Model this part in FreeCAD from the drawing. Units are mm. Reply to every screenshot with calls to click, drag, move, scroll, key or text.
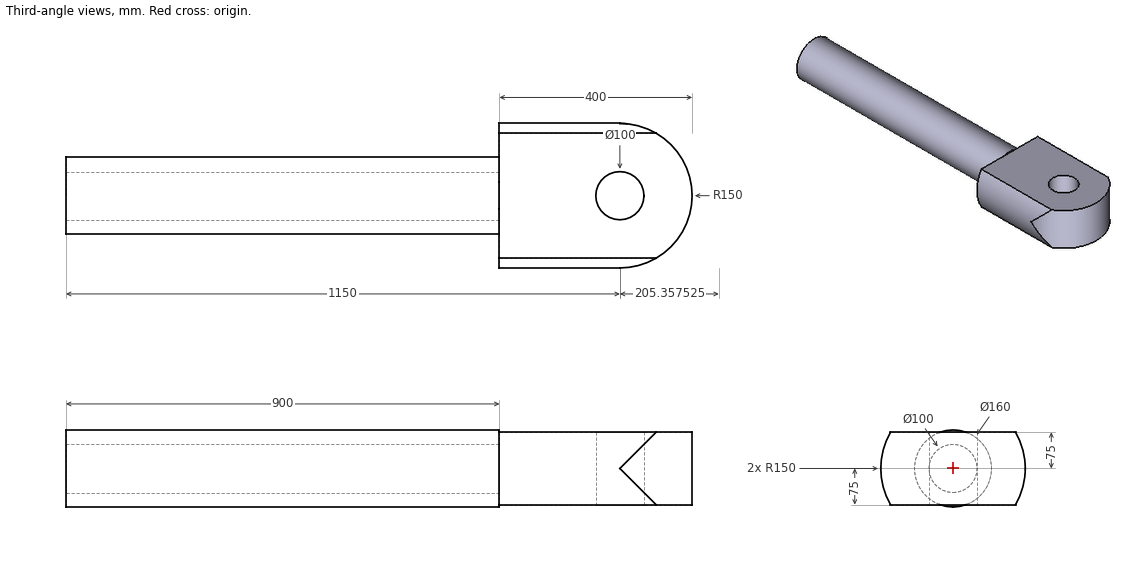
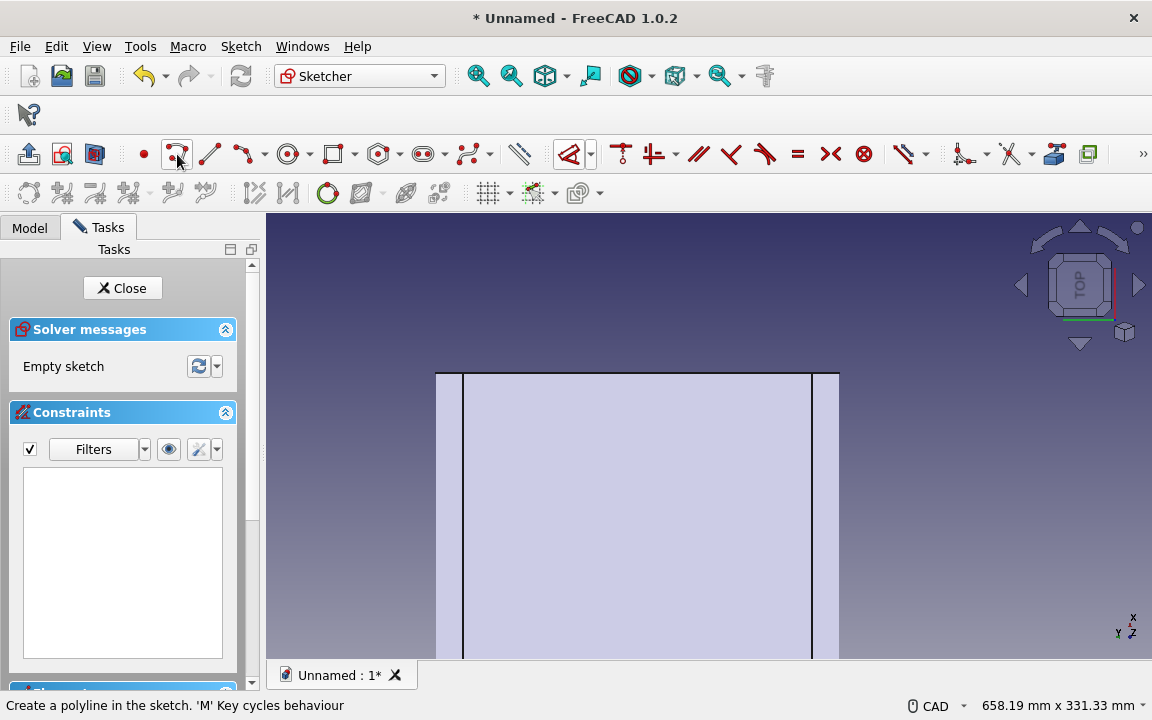
click(839, 575)
click(839, 299)
click(436, 299)
click(436, 575)
right_click(436, 575)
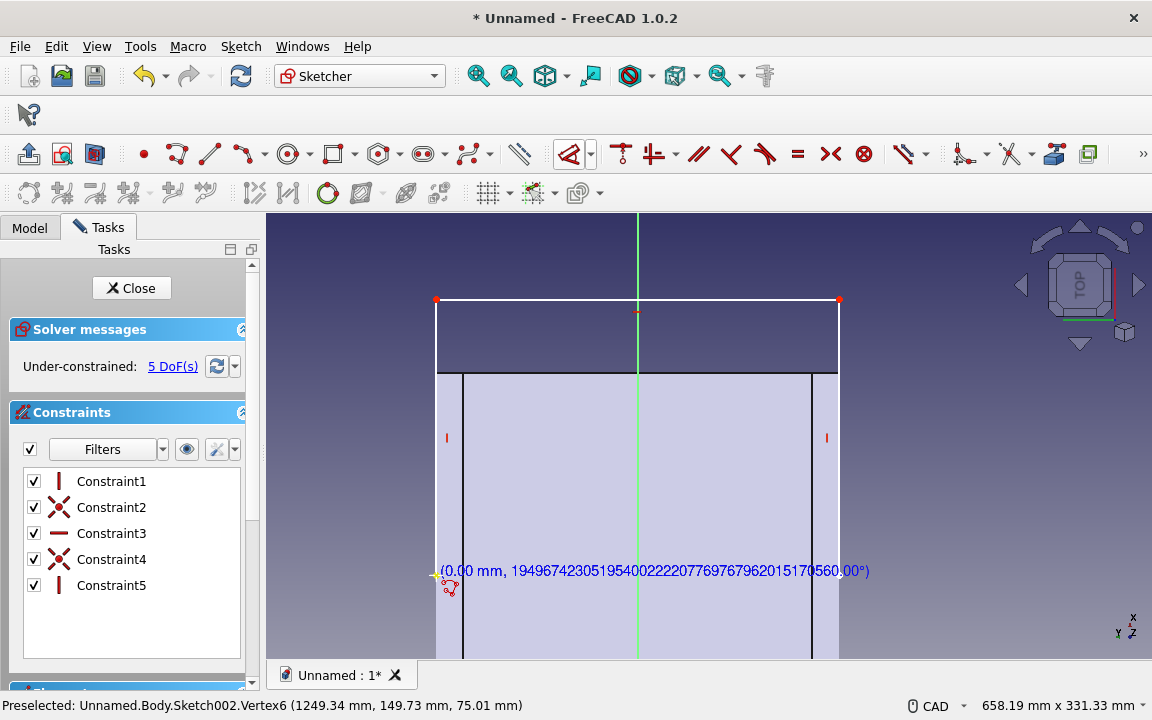
key(g)
key(3)
key(a)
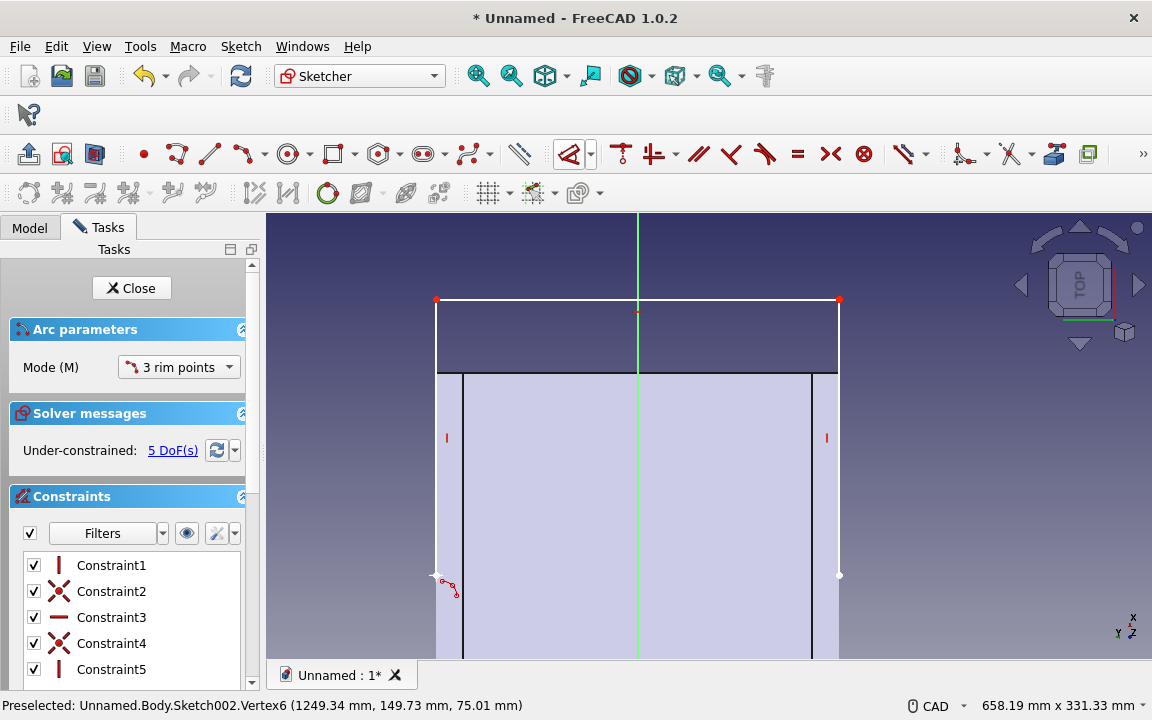
click(436, 576)
click(839, 576)
click(700, 383)
key(Escape)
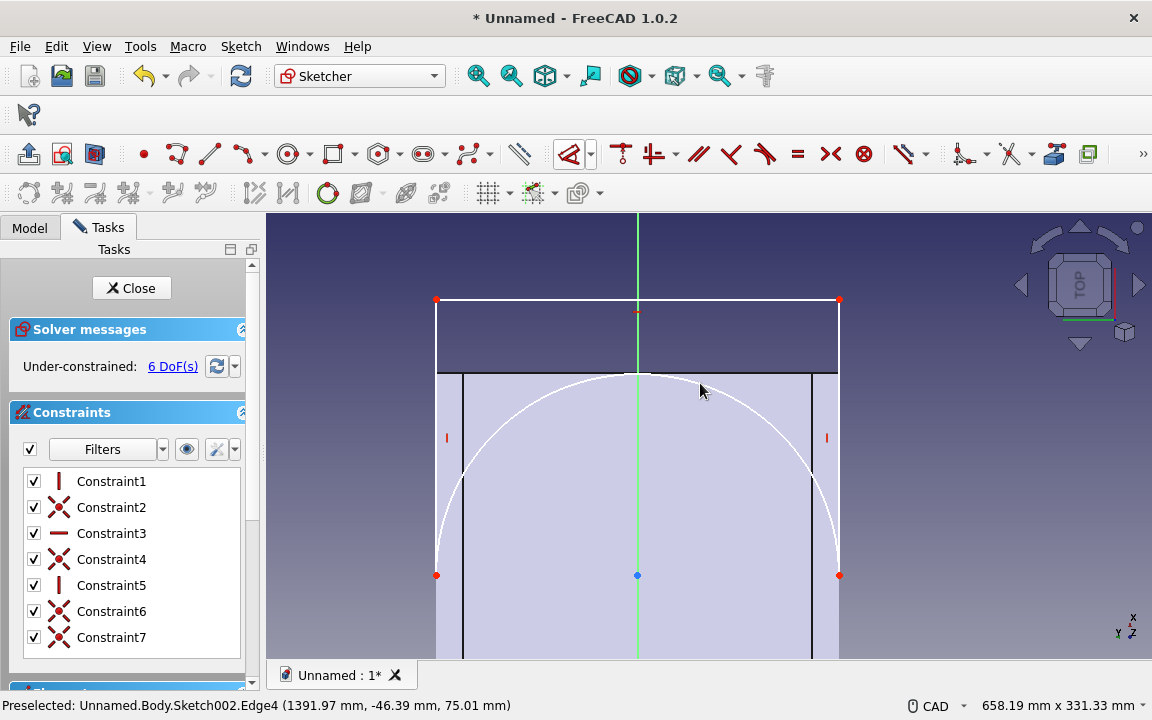
click(638, 576)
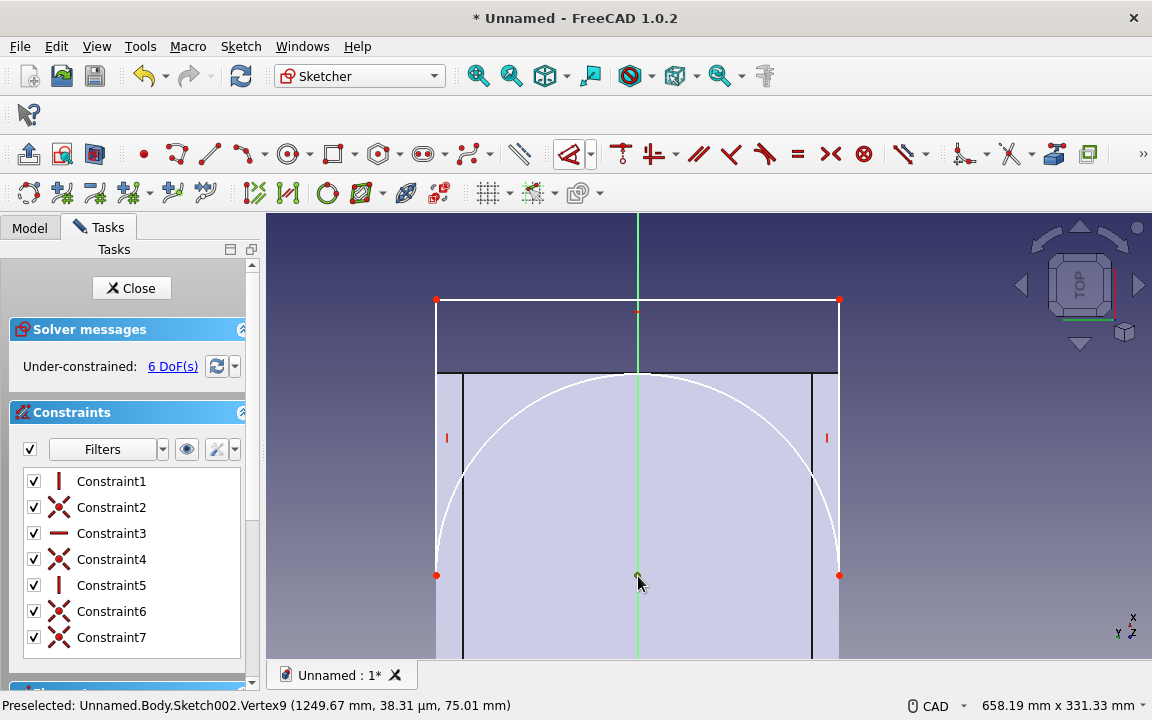
click(638, 603)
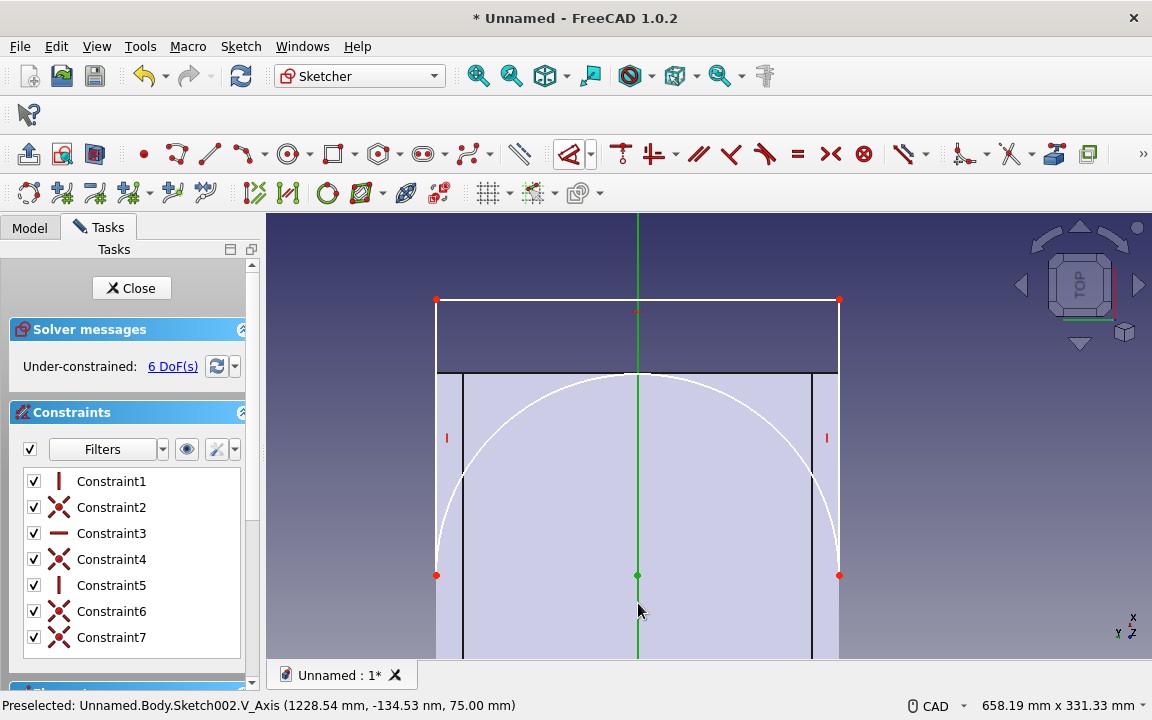
key(c)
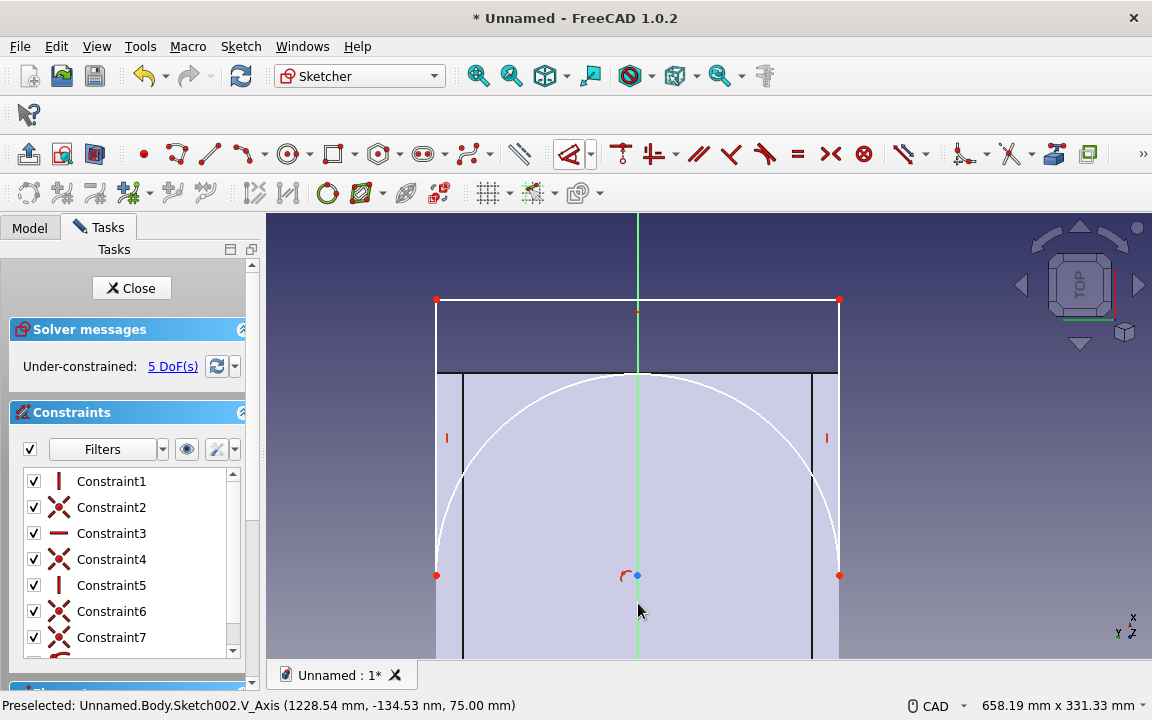
click(568, 154)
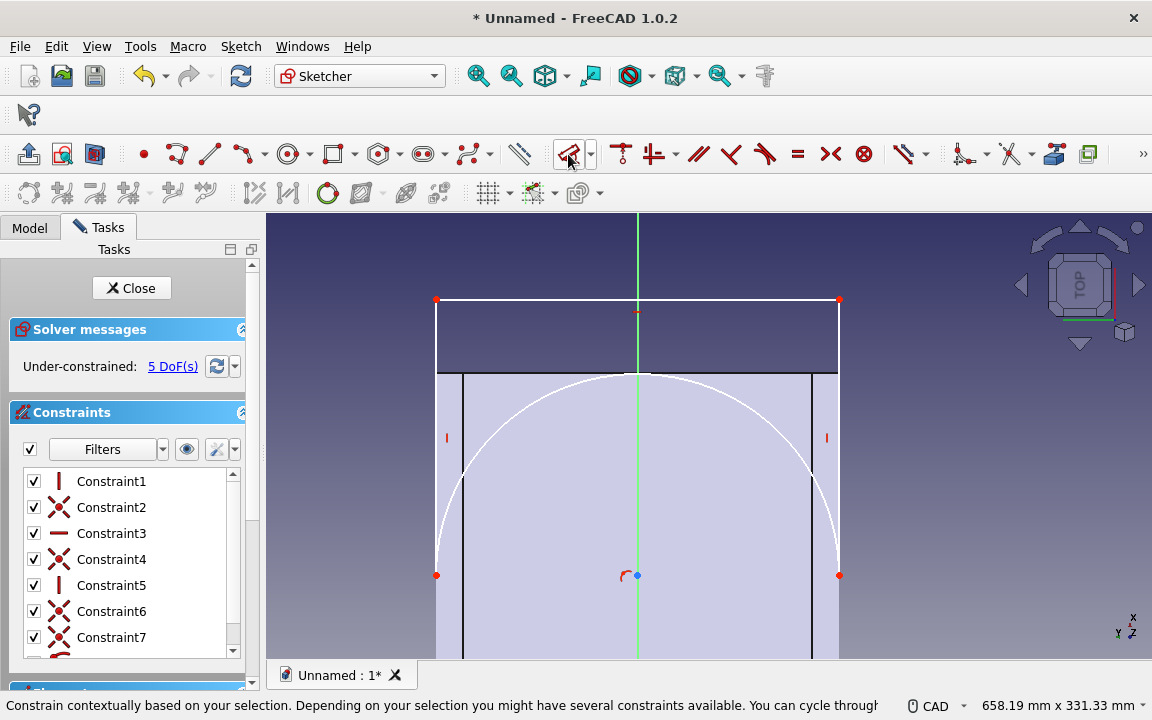
click(756, 413)
click(775, 387)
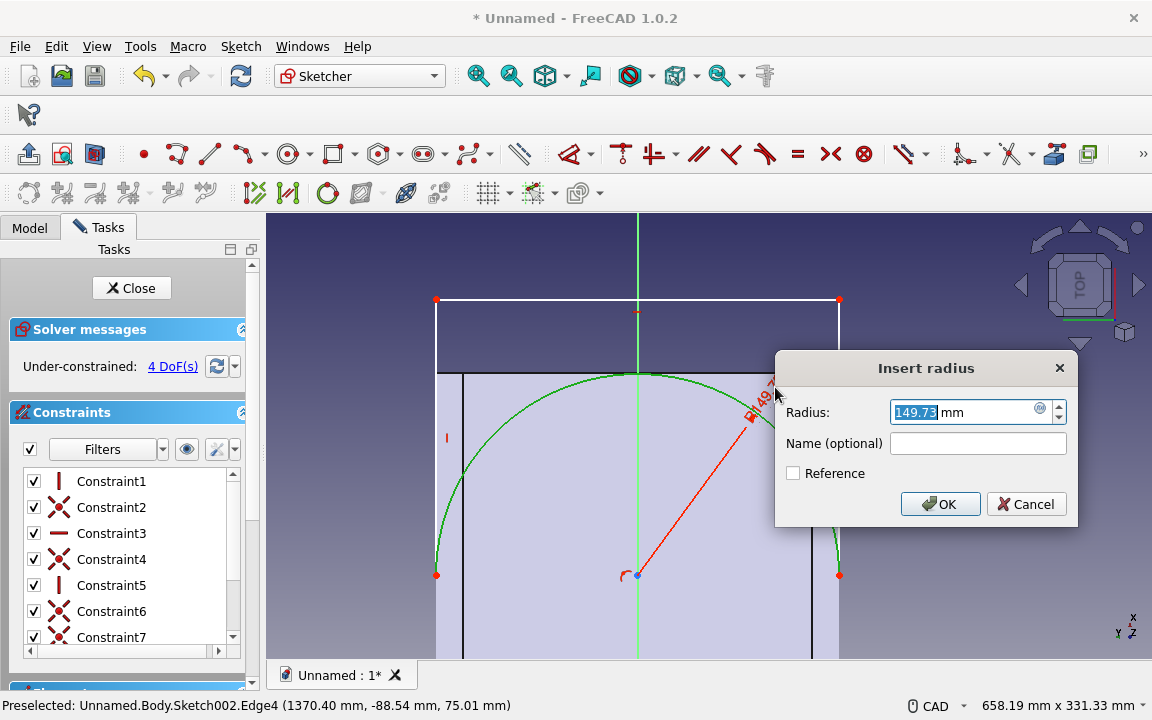
text(150)
key(Return)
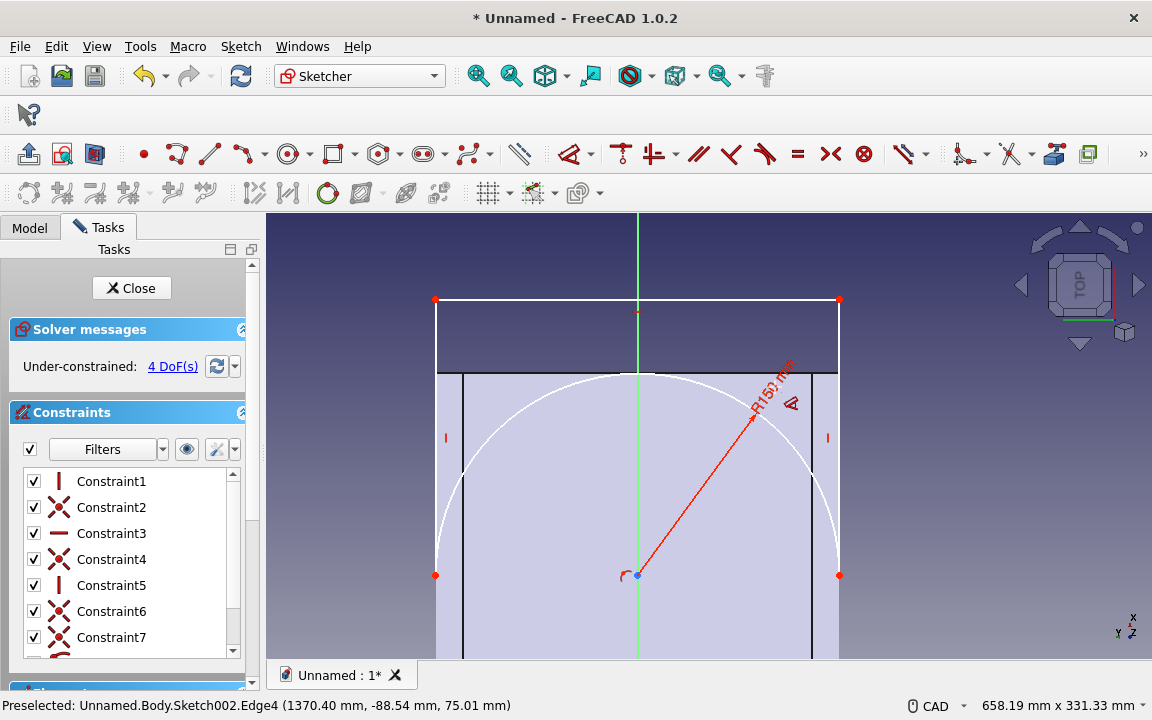
click(839, 576)
click(873, 603)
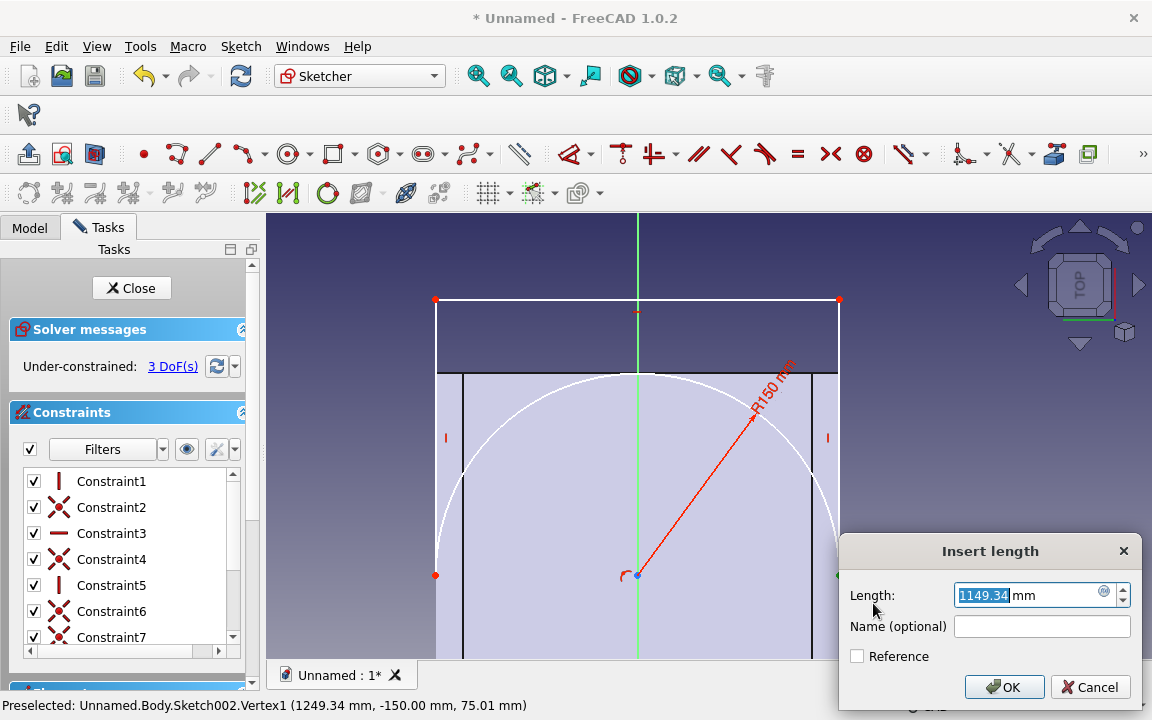
text(1150)
key(Return)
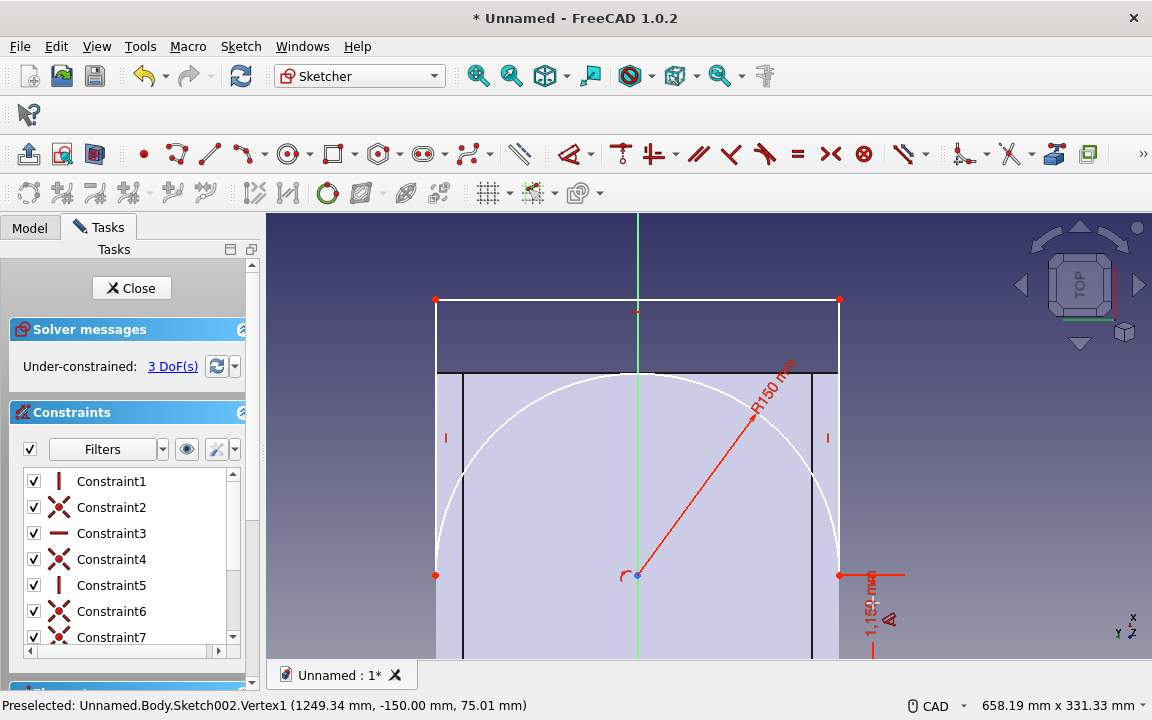
click(436, 576)
click(402, 604)